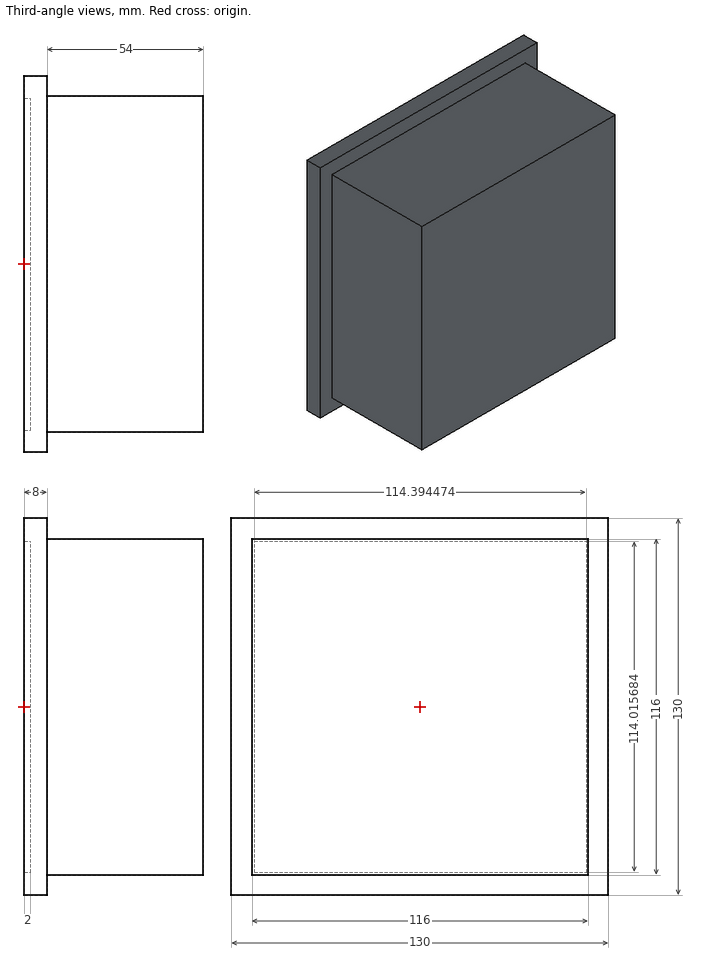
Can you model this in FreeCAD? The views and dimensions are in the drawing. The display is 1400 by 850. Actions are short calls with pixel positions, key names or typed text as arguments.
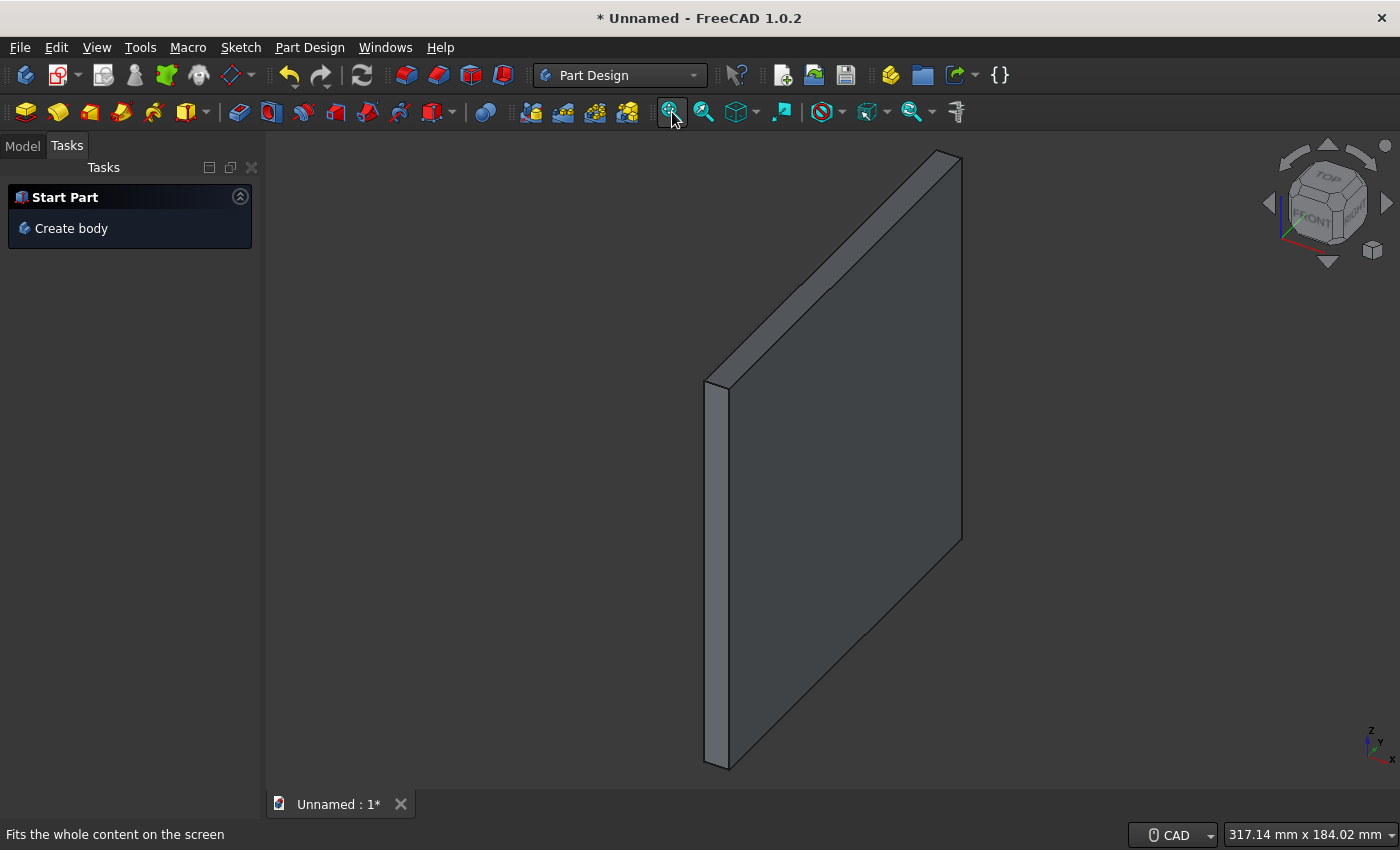
click(845, 463)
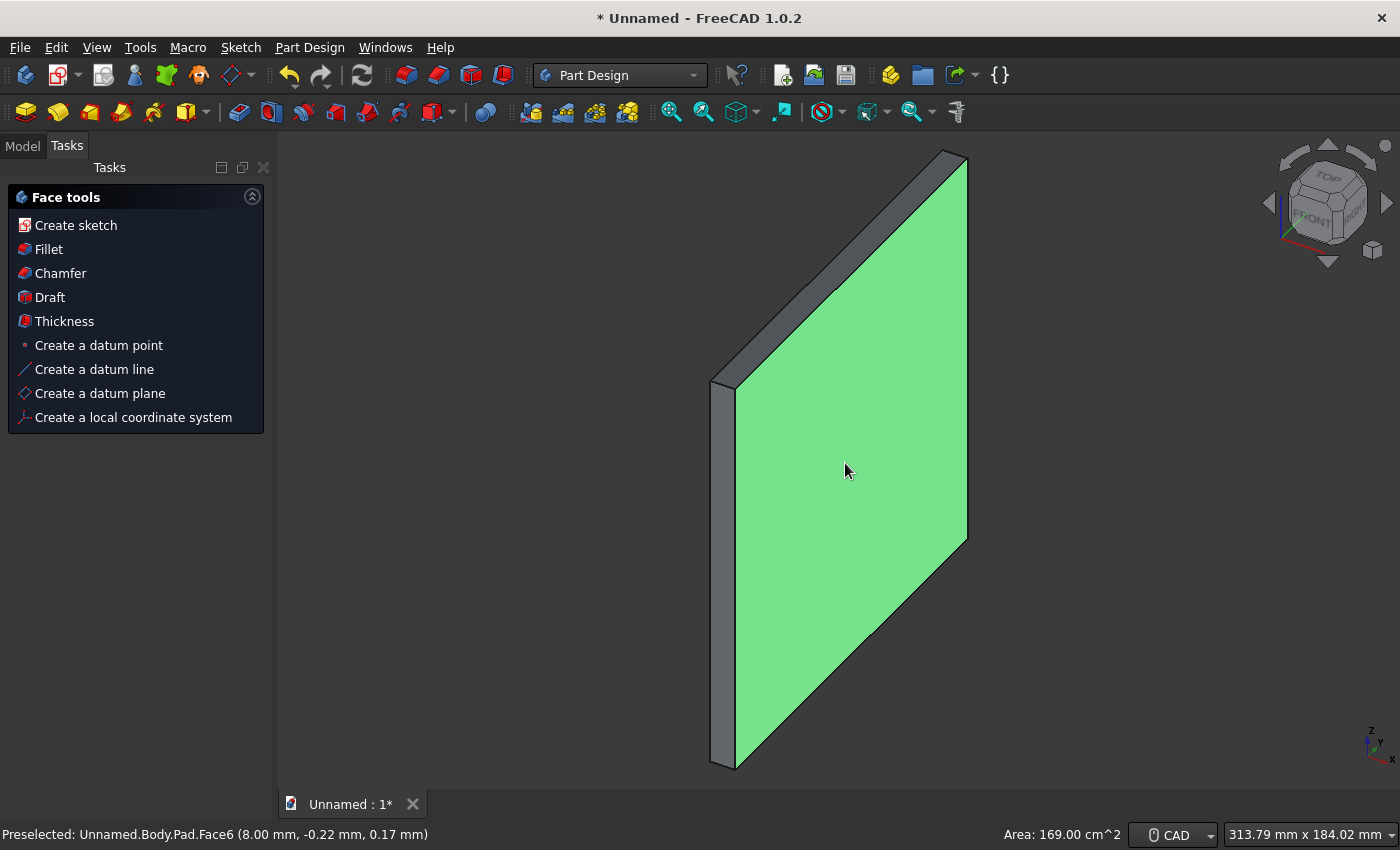
click(58, 76)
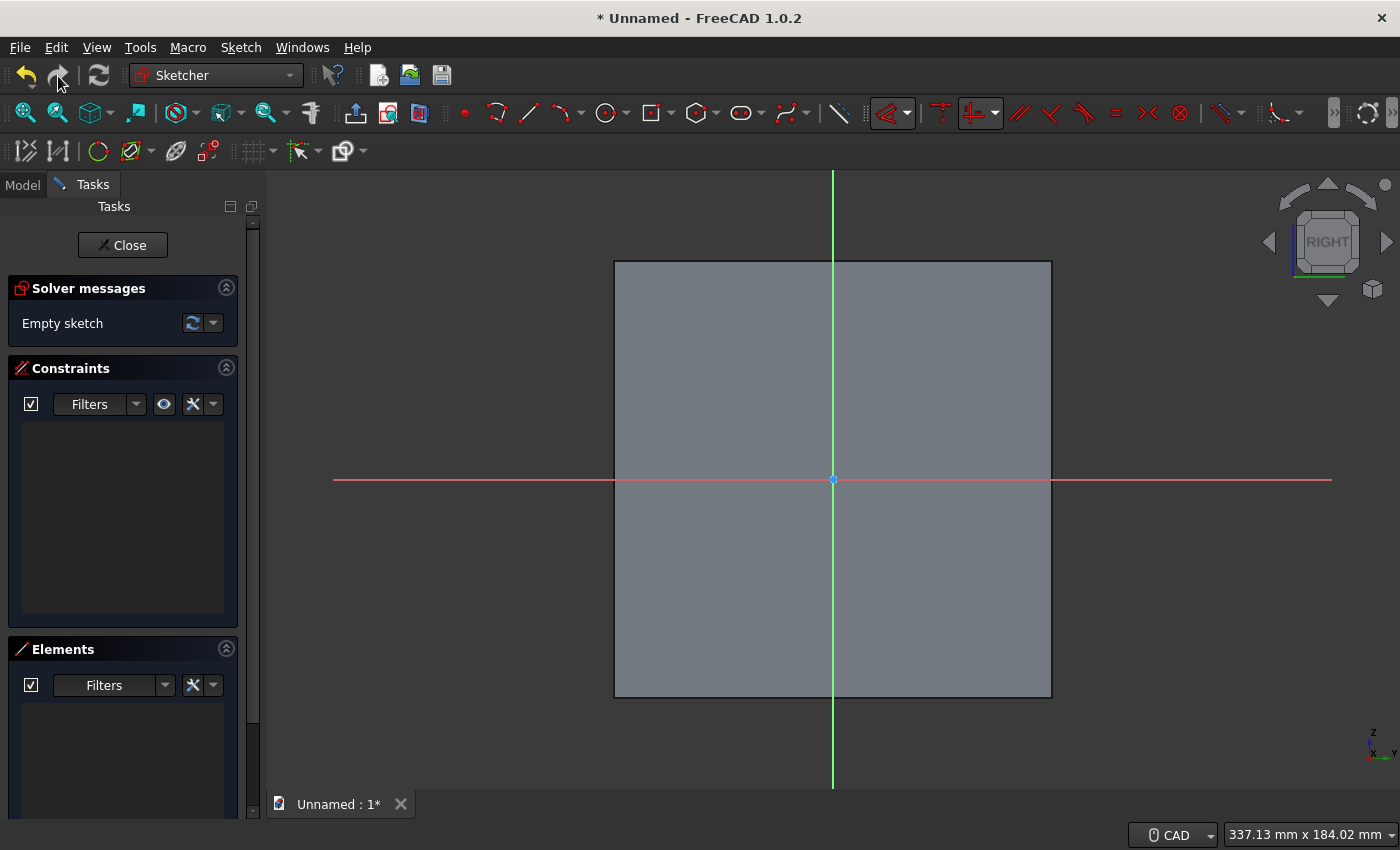
click(652, 114)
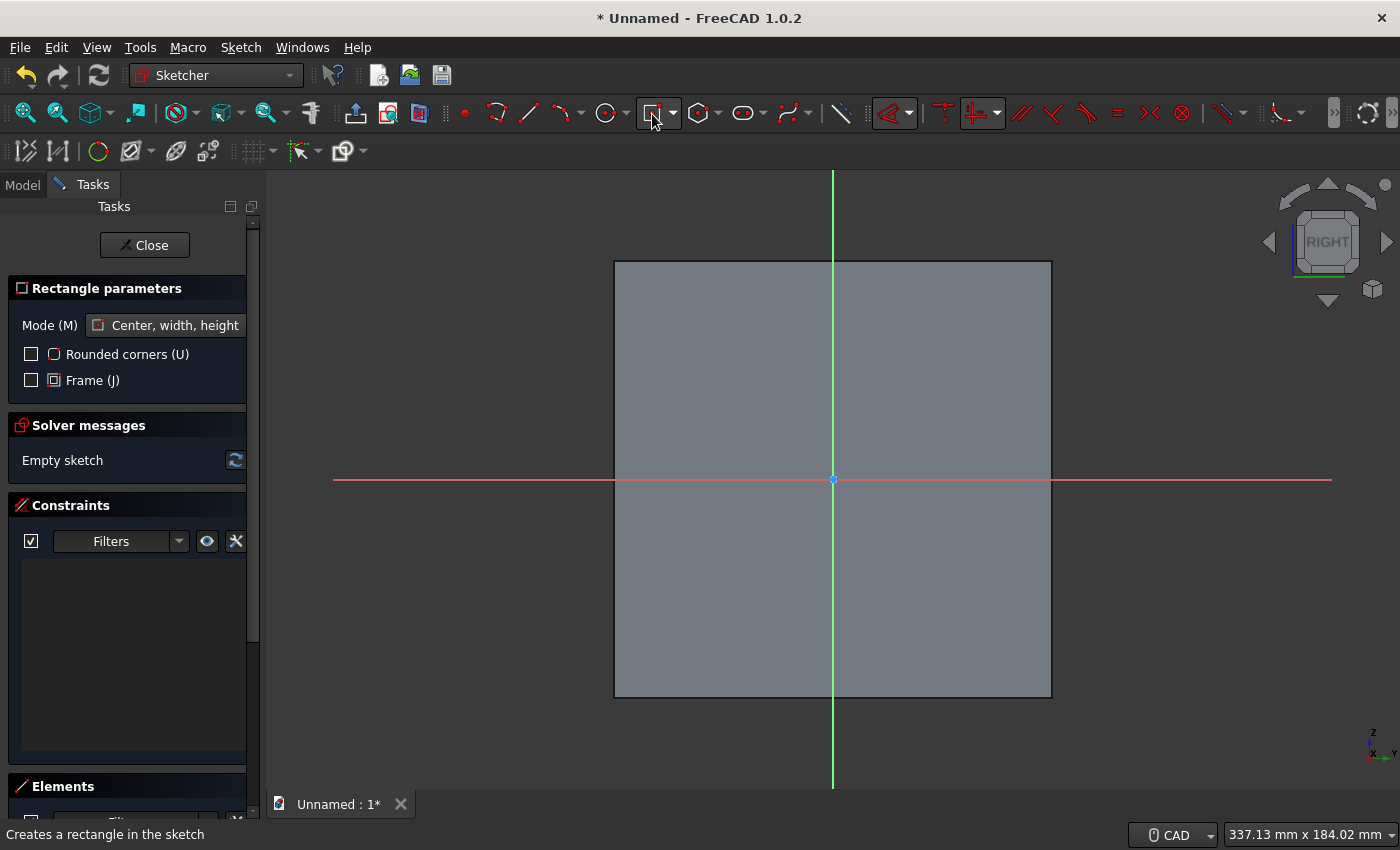
click(833, 480)
click(1028, 284)
key(Escape)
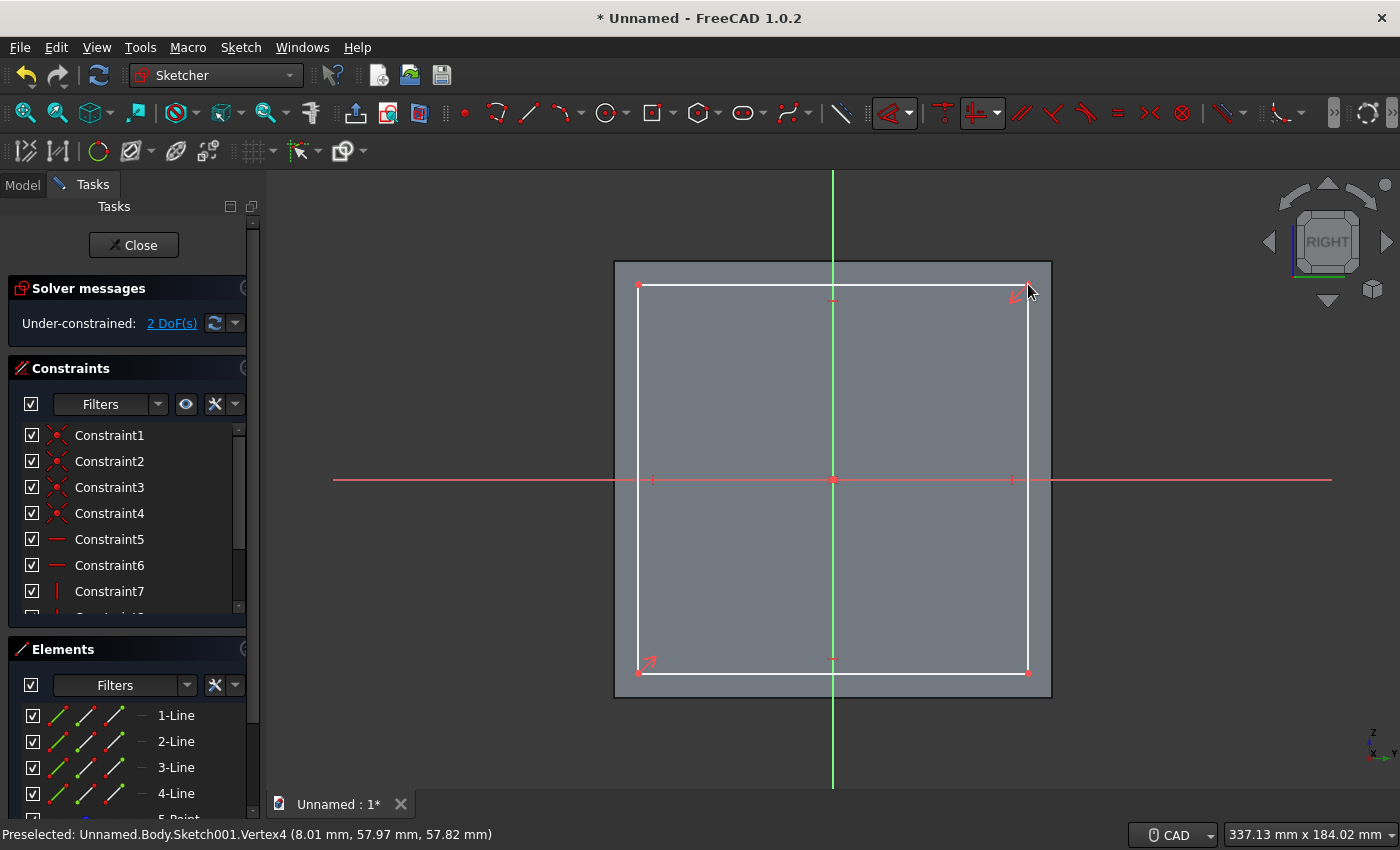
click(755, 674)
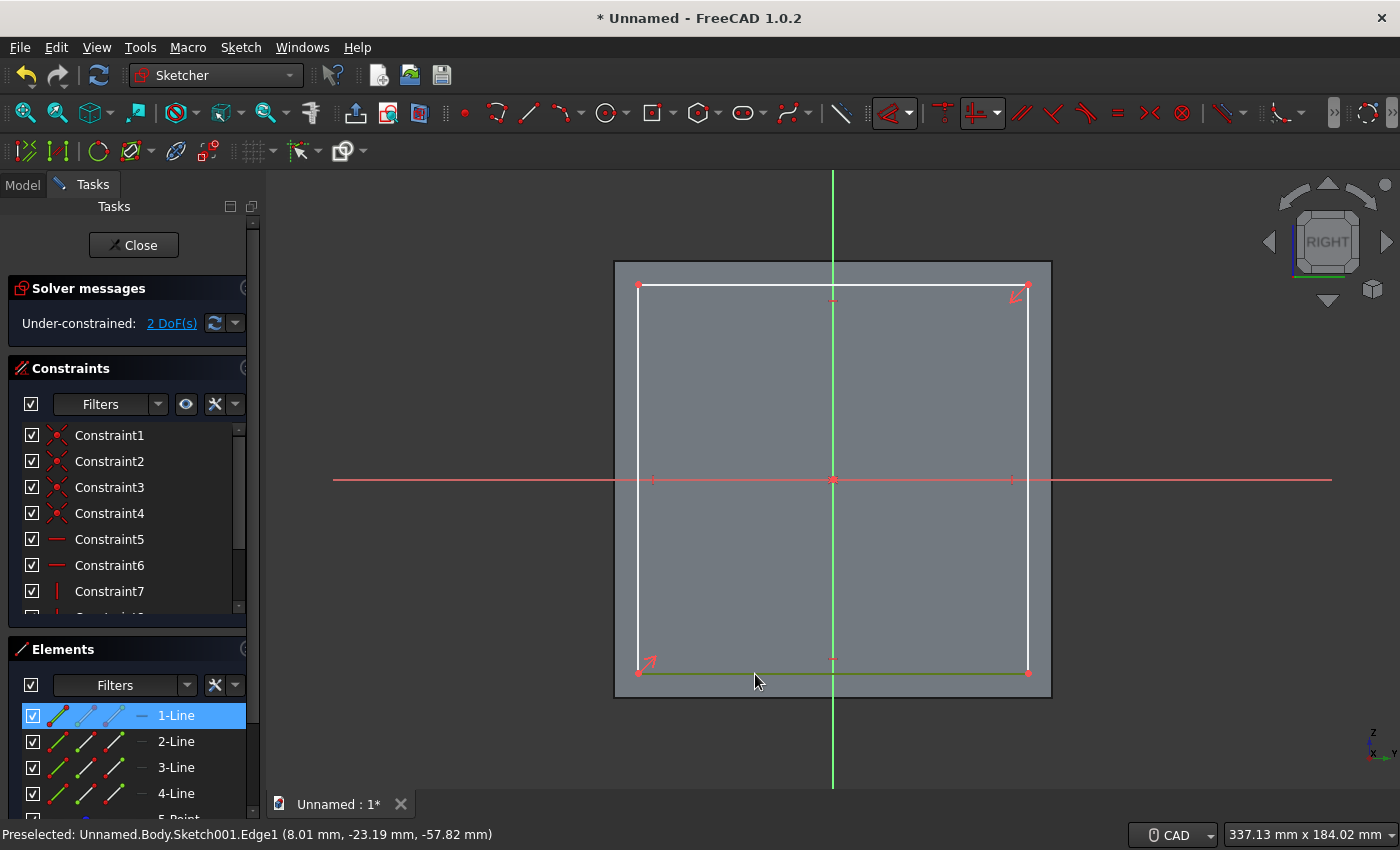
click(912, 114)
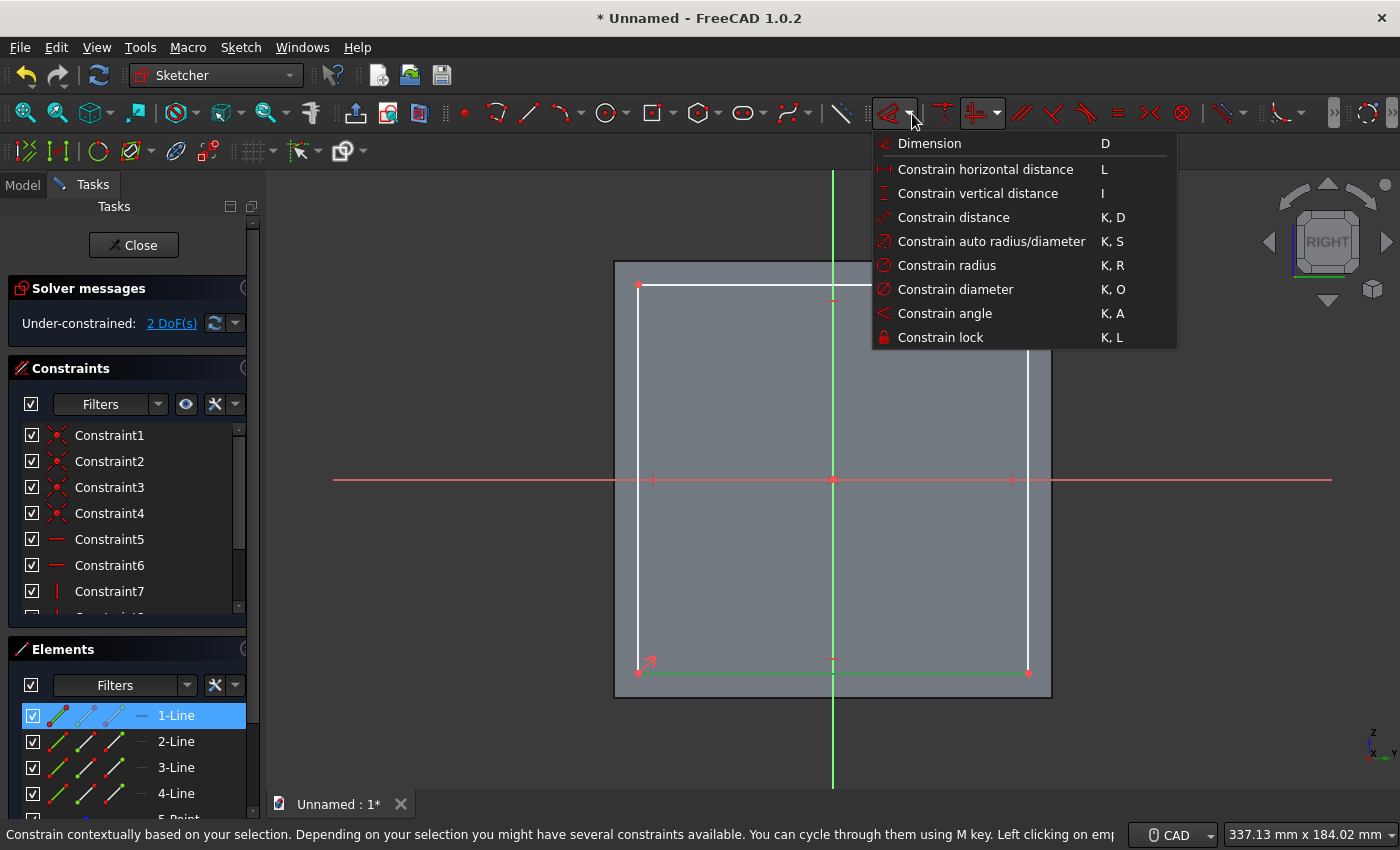
click(1025, 169)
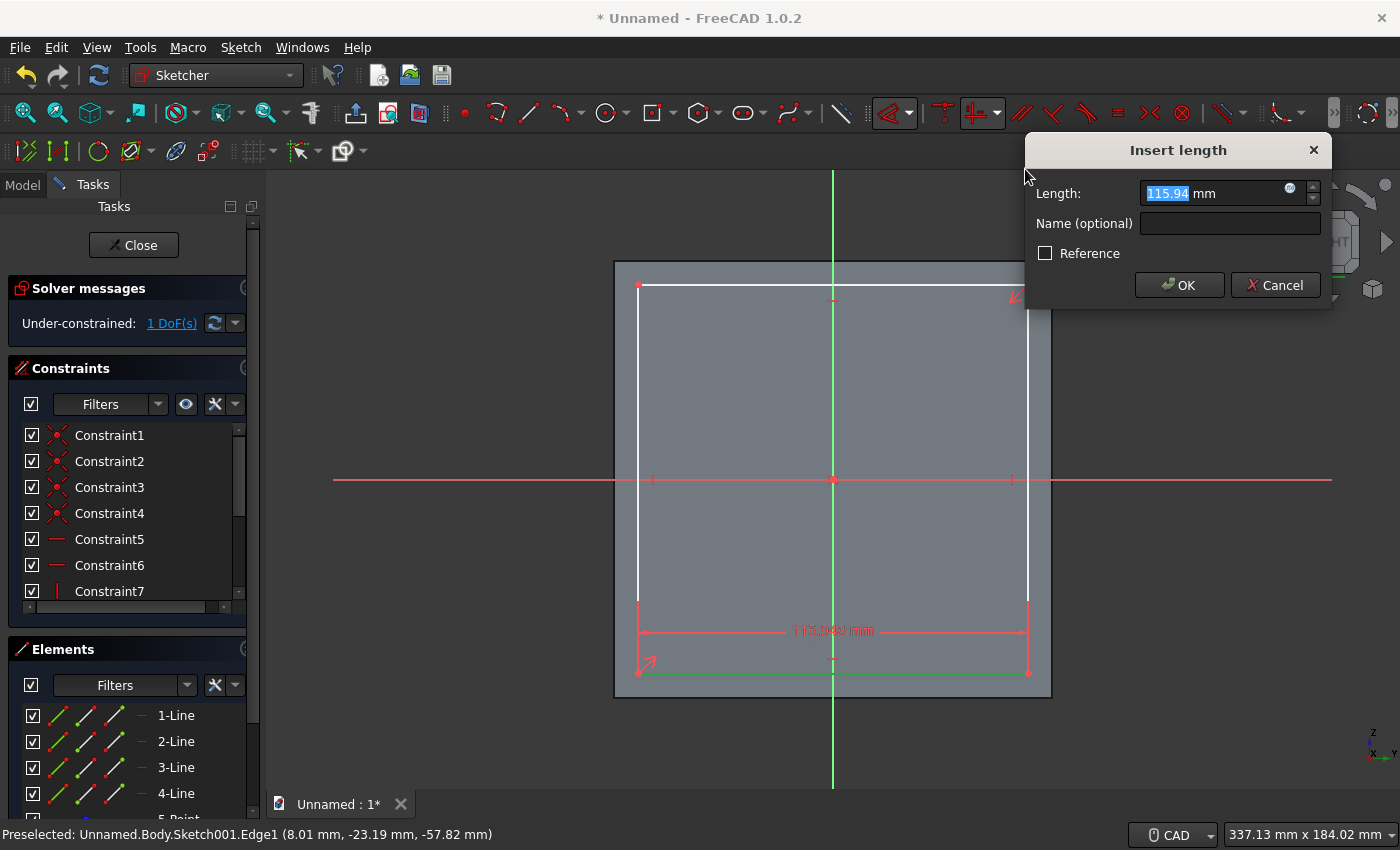
text(116)
key(Return)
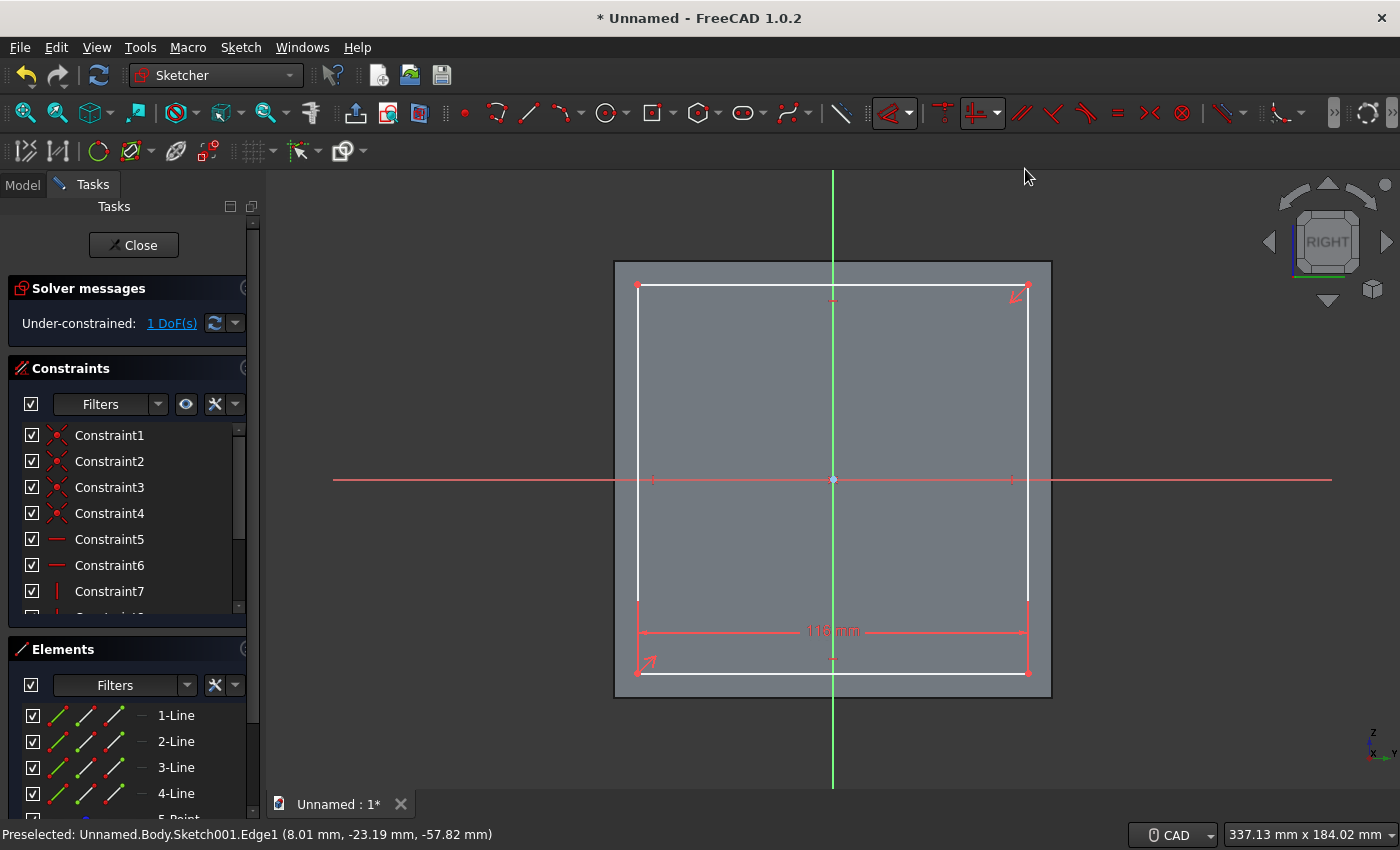
click(1028, 557)